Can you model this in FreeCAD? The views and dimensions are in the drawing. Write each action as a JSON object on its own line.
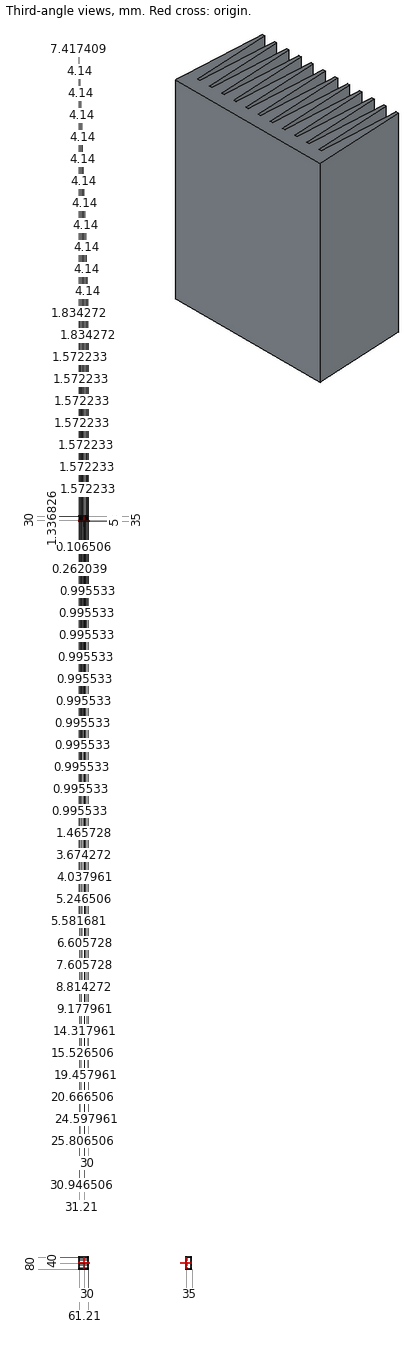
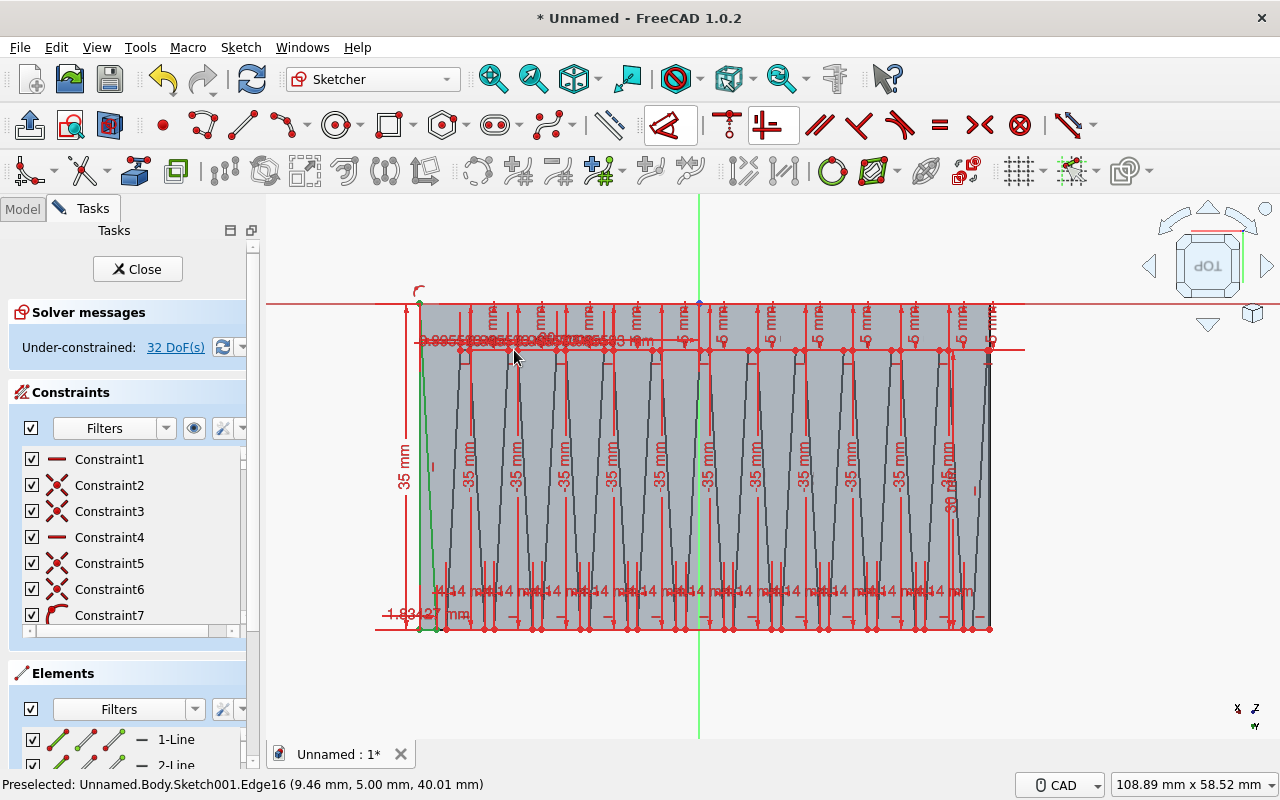
{"action": "scroll", "coordinate": [658, 350], "scroll_direction": "up", "scroll_amount": 9}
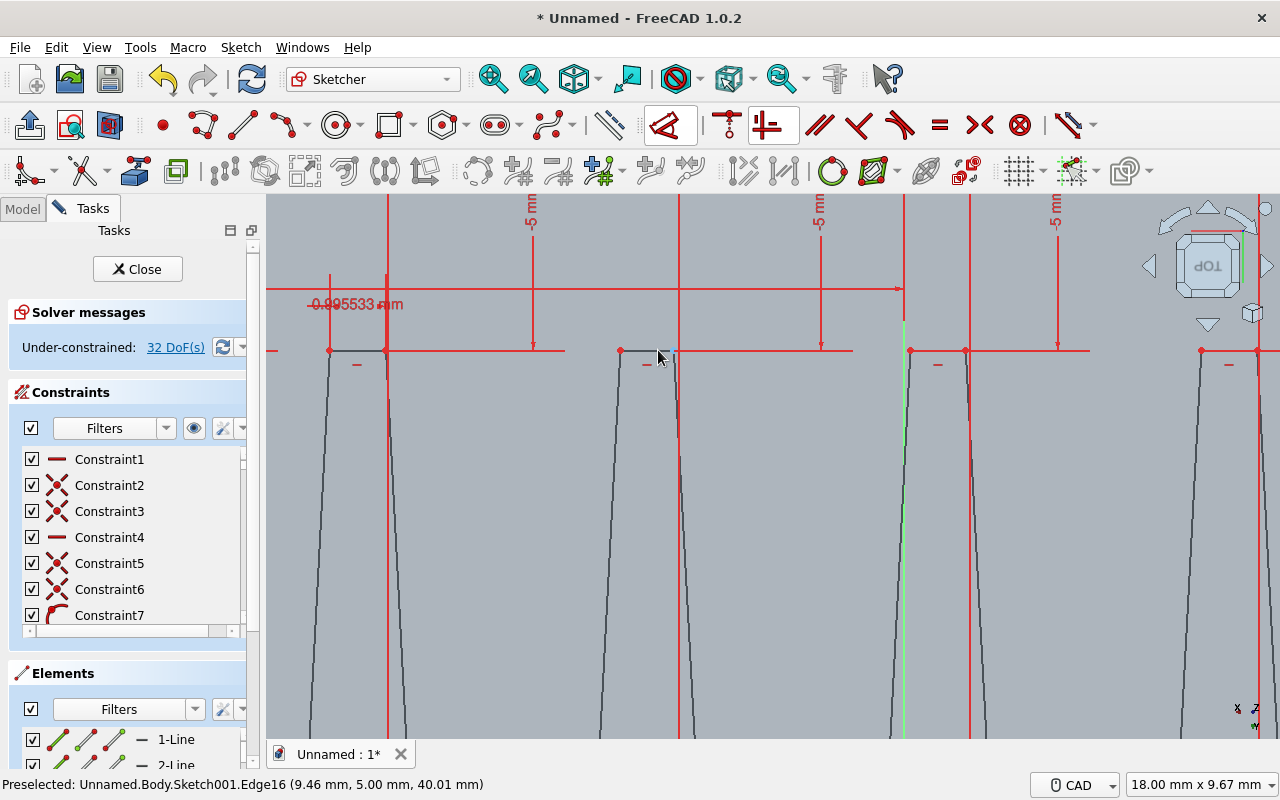
{"action": "left_click", "coordinate": [658, 351]}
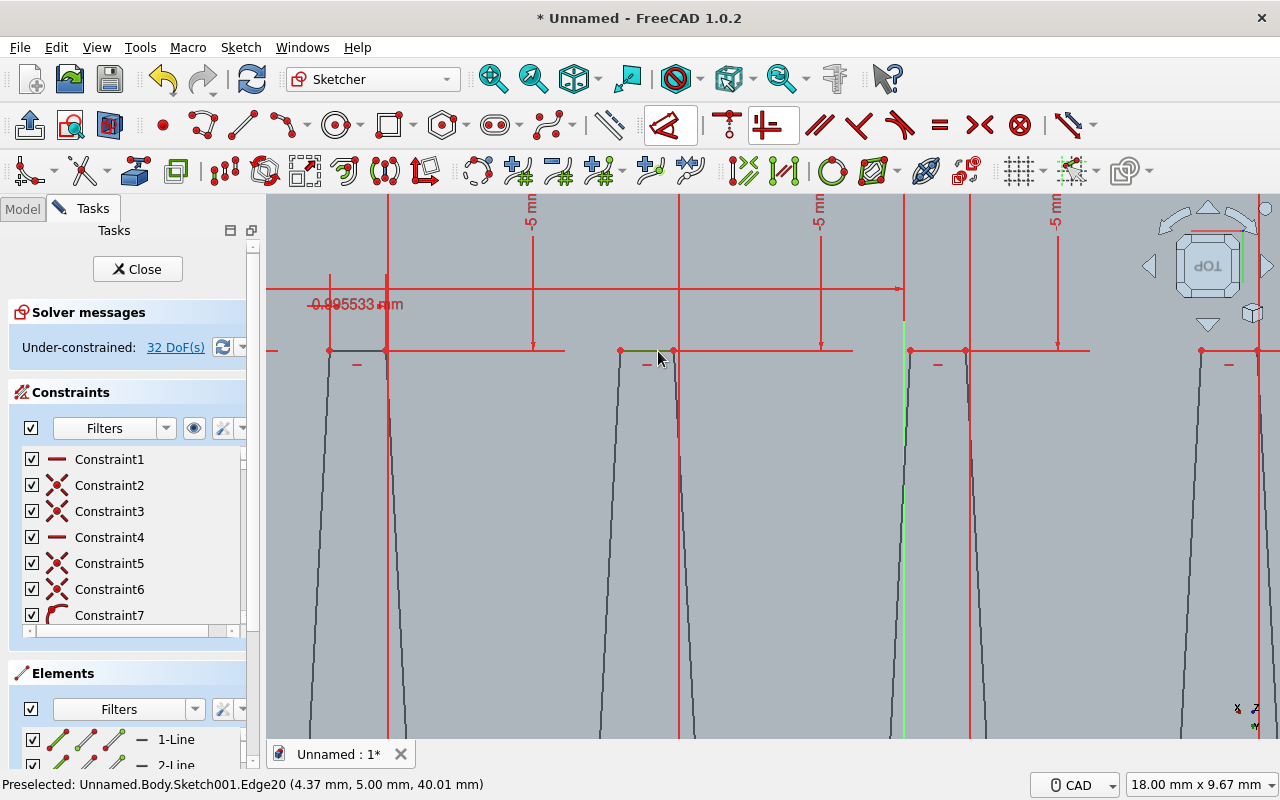
{"action": "key", "text": "l"}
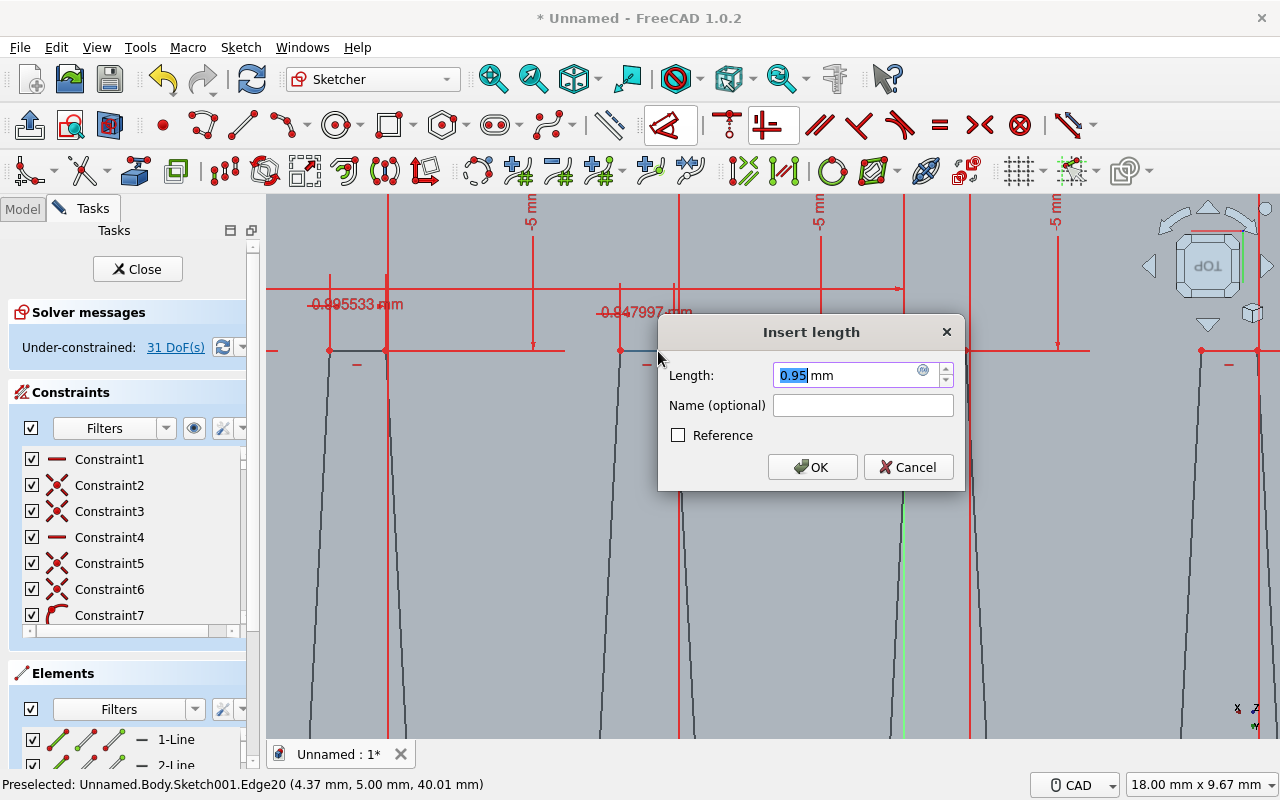
{"action": "type", "text": "0.995533"}
{"action": "key", "text": "Return"}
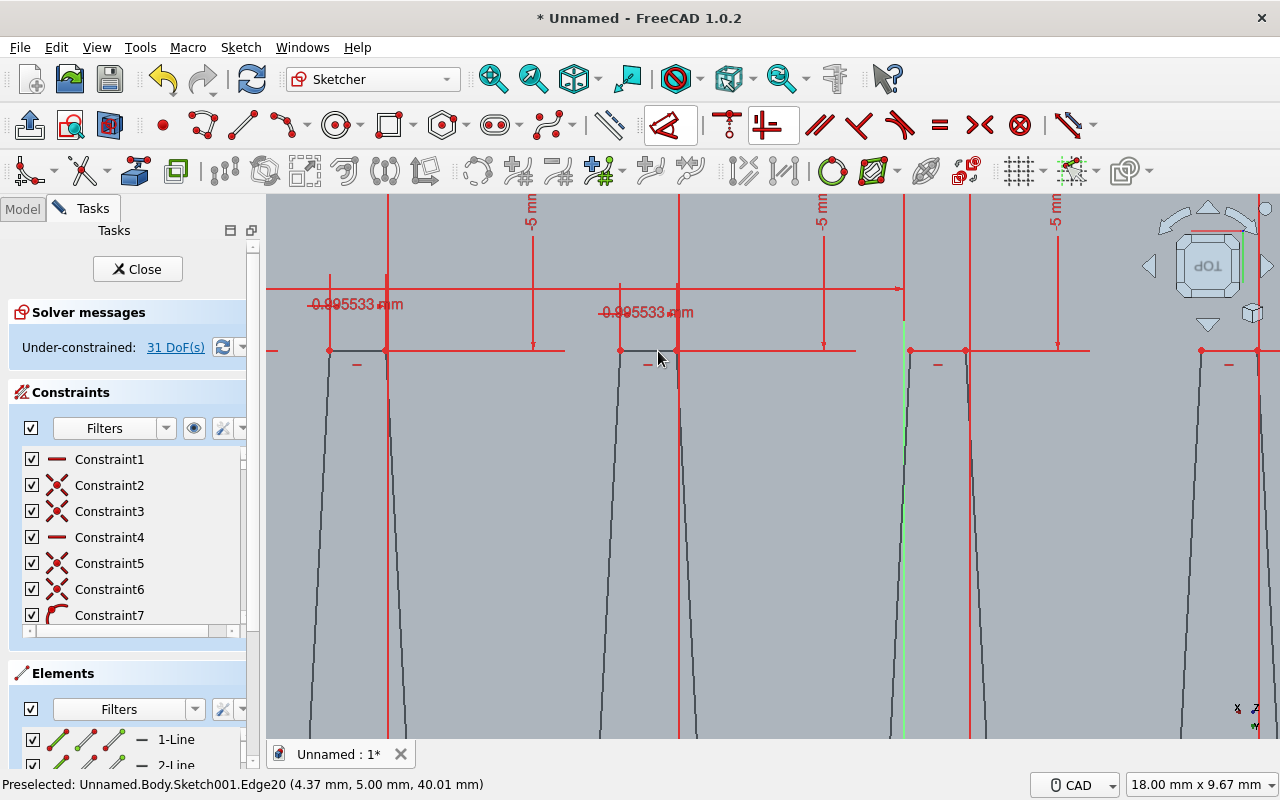
{"action": "left_click", "coordinate": [949, 351]}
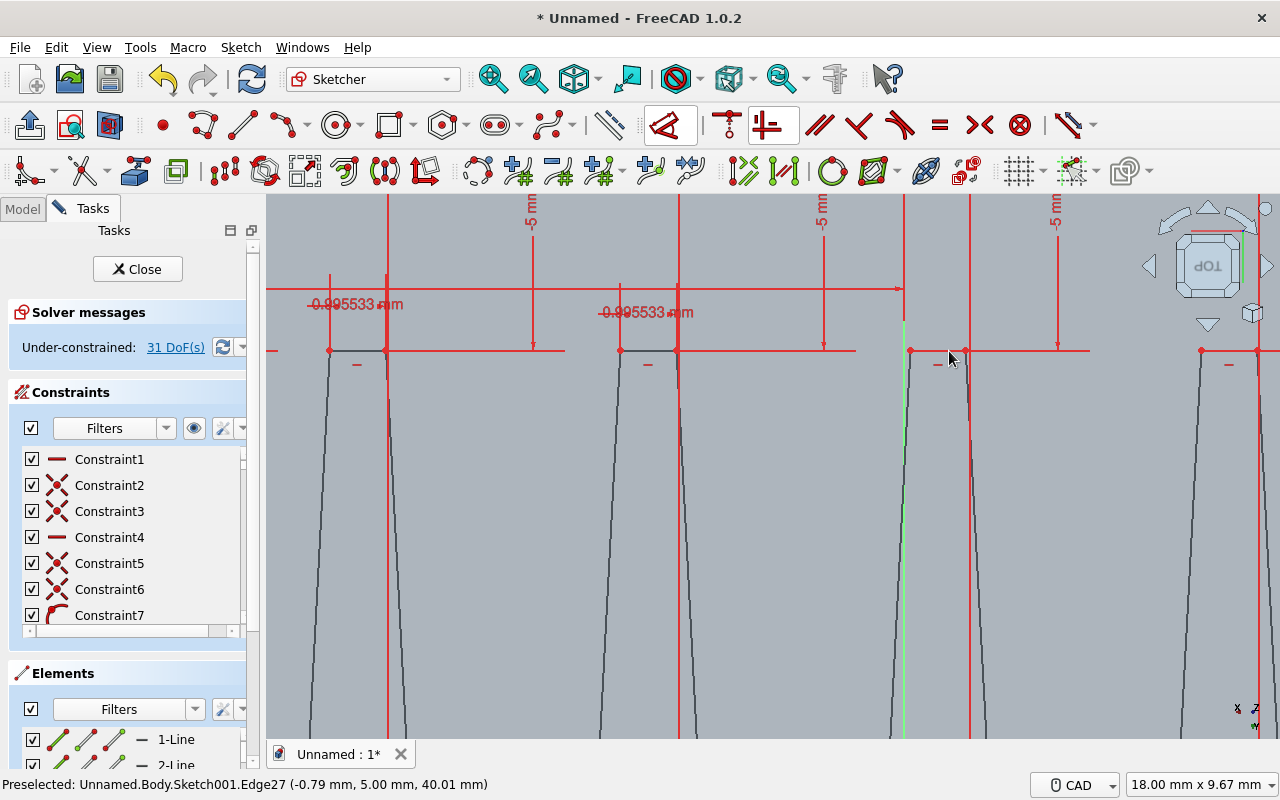
{"action": "left_click", "coordinate": [692, 126]}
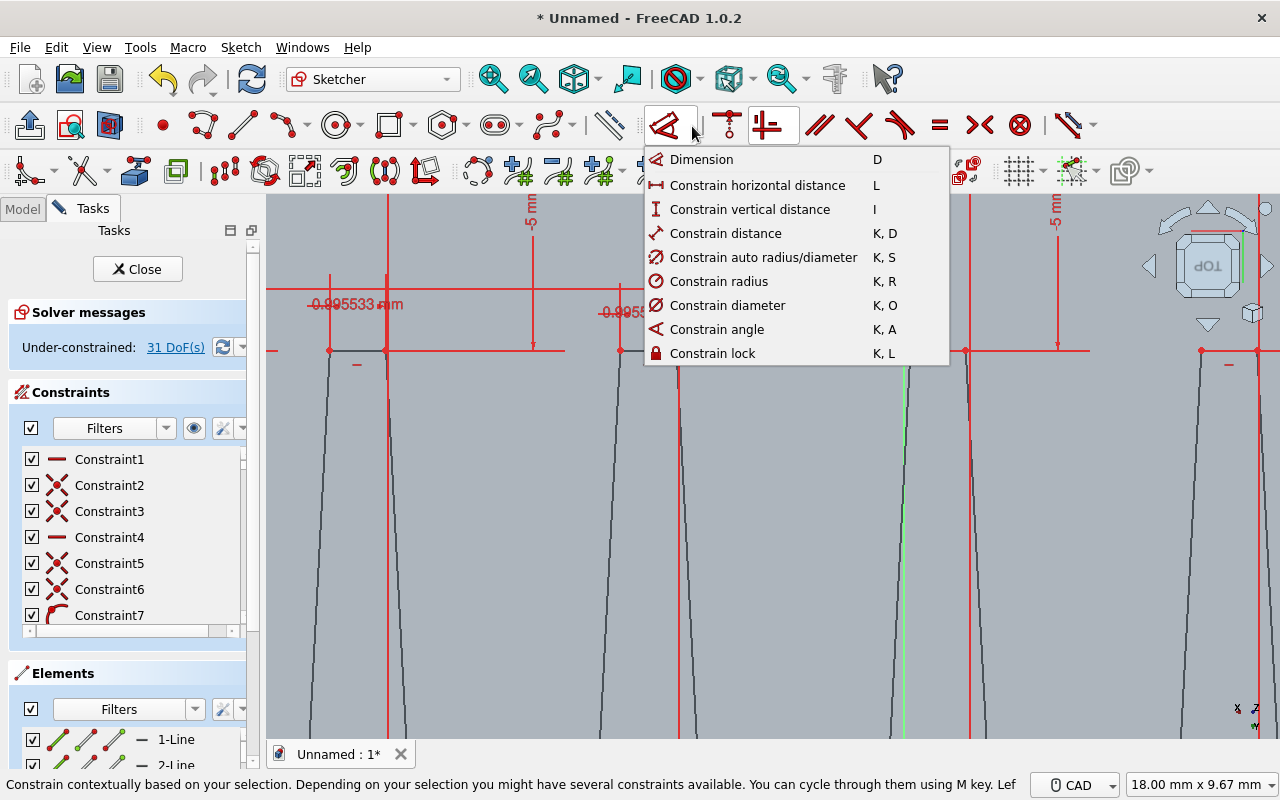
{"action": "left_click", "coordinate": [797, 185]}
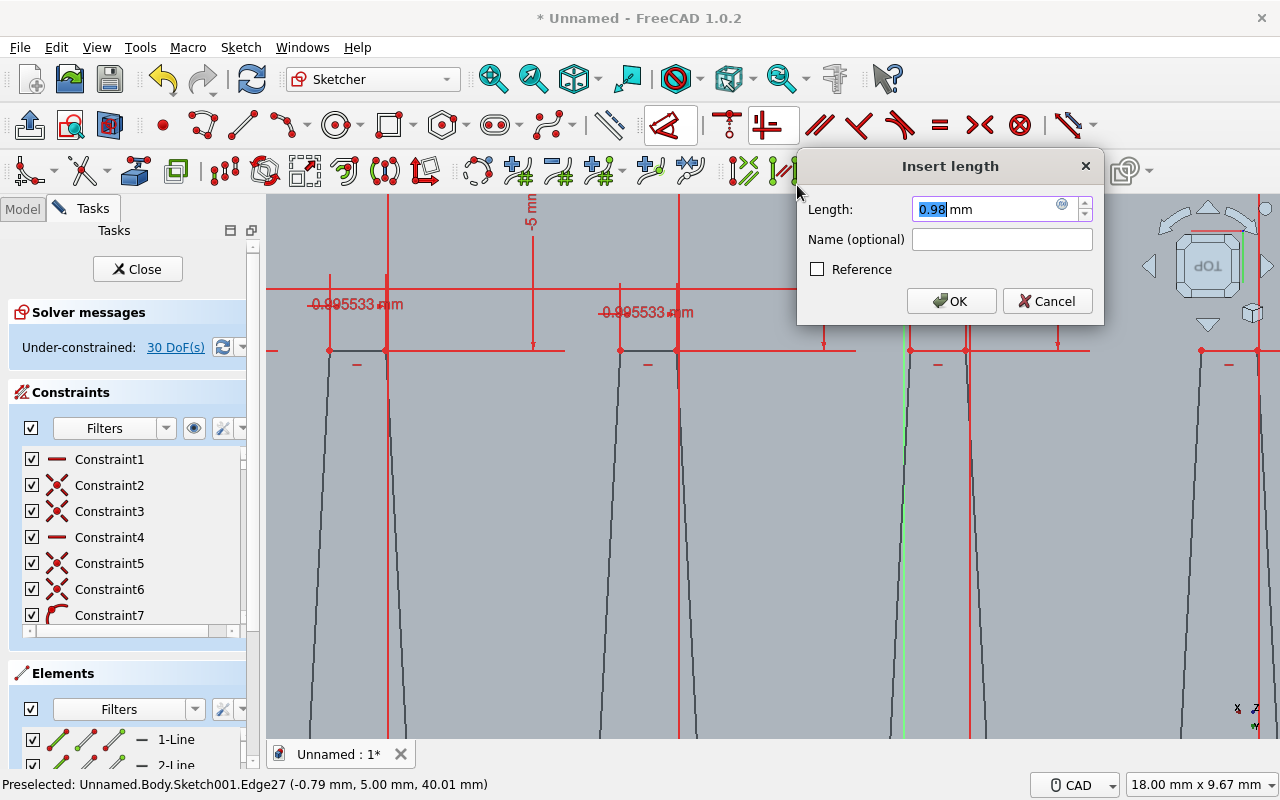
{"action": "type", "text": "0.995533"}
{"action": "key", "text": "Return"}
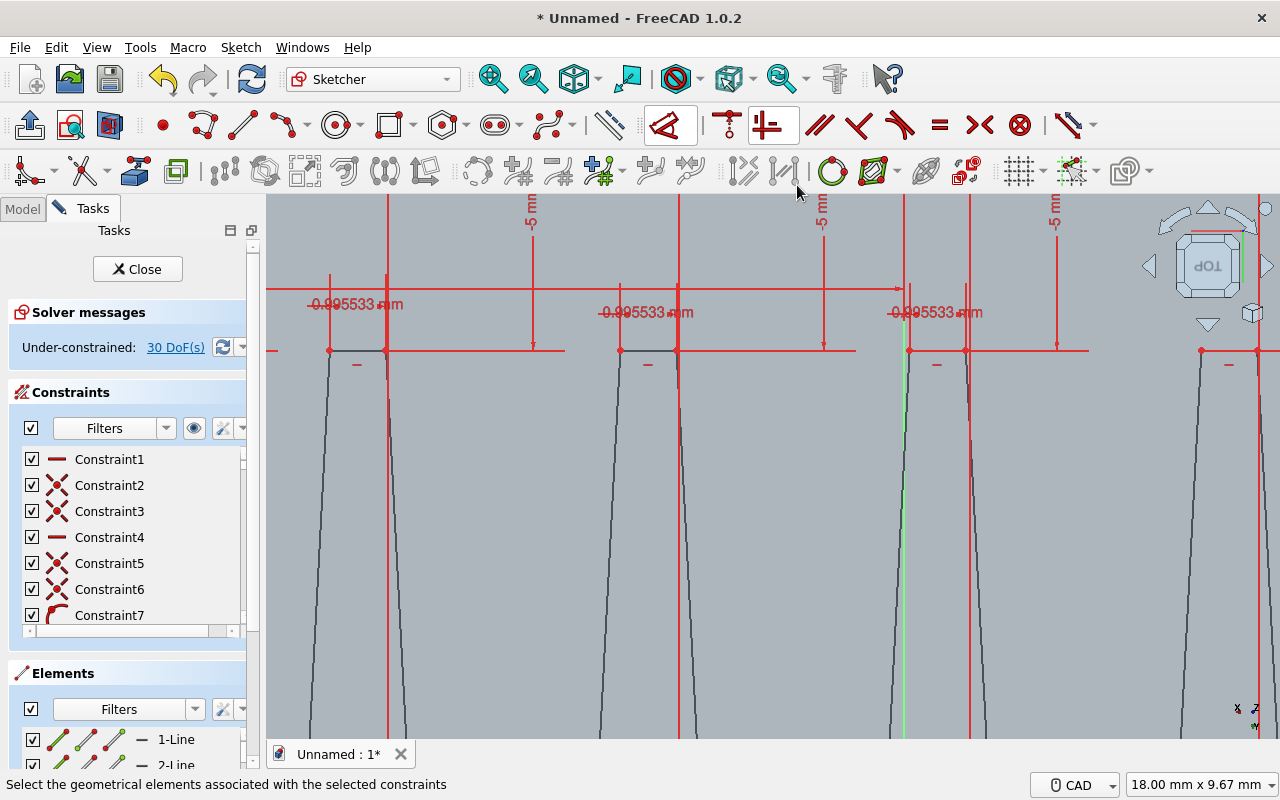
{"action": "scroll", "coordinate": [658, 350], "scroll_direction": "down", "scroll_amount": 9}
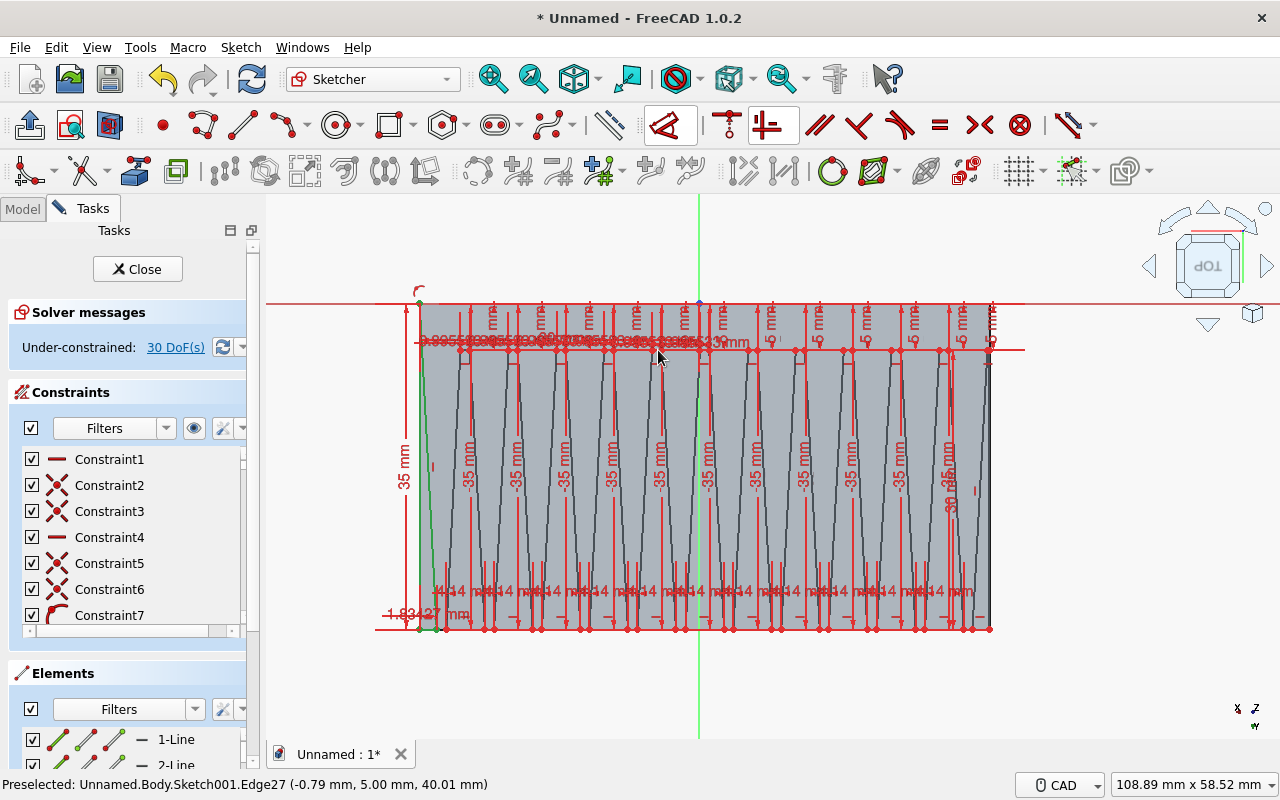
{"action": "scroll", "coordinate": [755, 350], "scroll_direction": "up", "scroll_amount": 9}